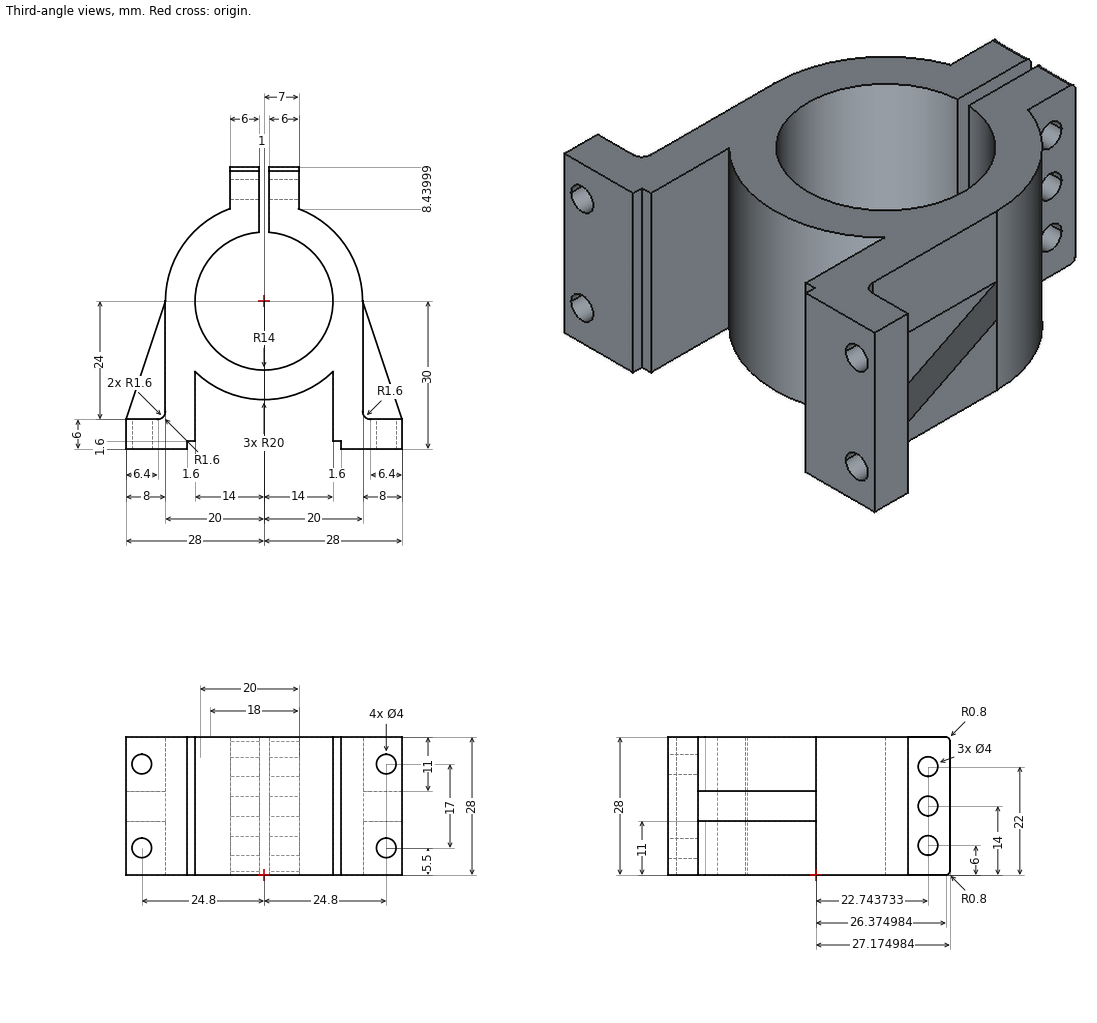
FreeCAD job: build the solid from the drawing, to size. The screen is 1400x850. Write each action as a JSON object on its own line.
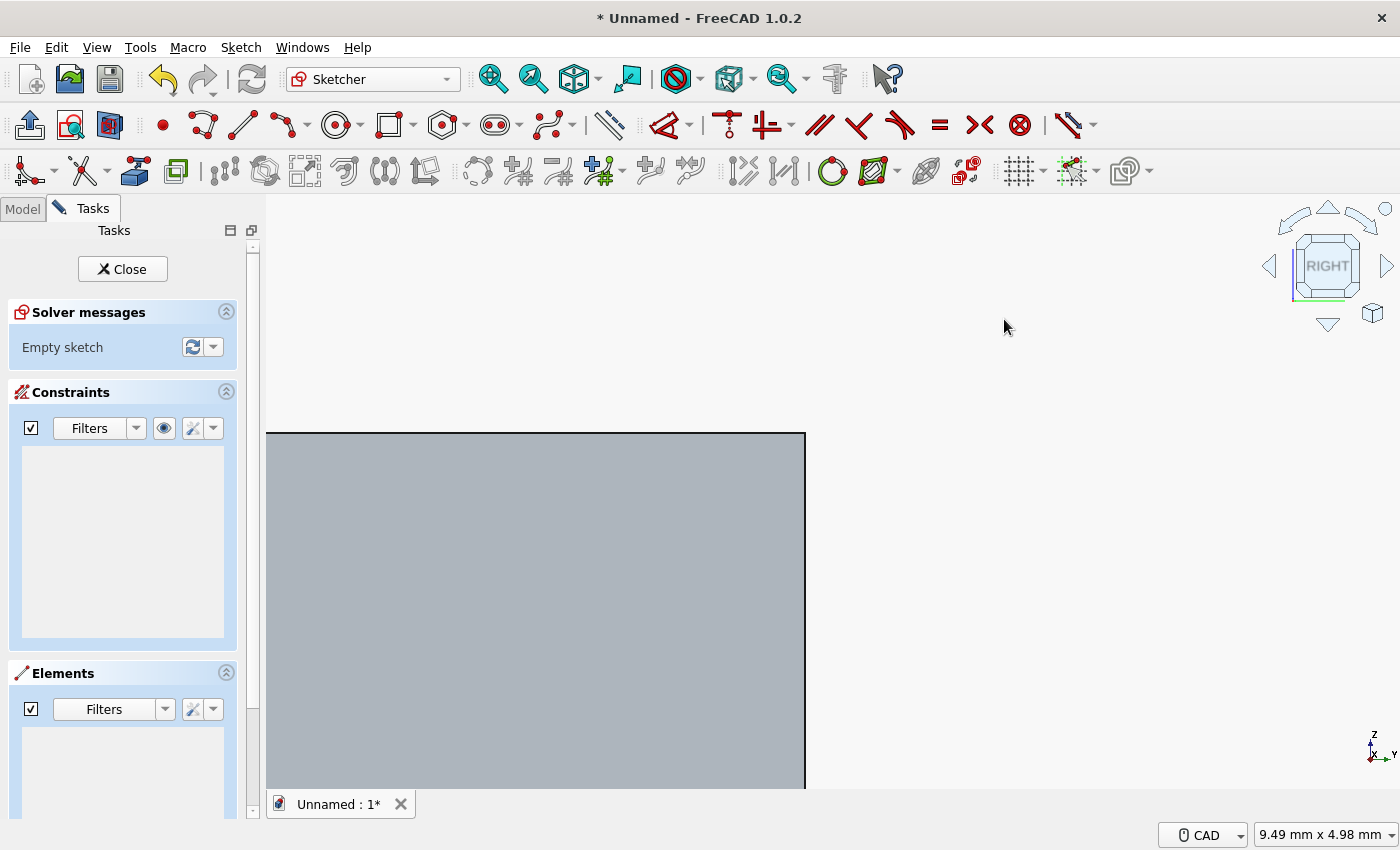
{"action": "scroll", "coordinate": [754, 478], "scroll_direction": "up", "scroll_amount": 7}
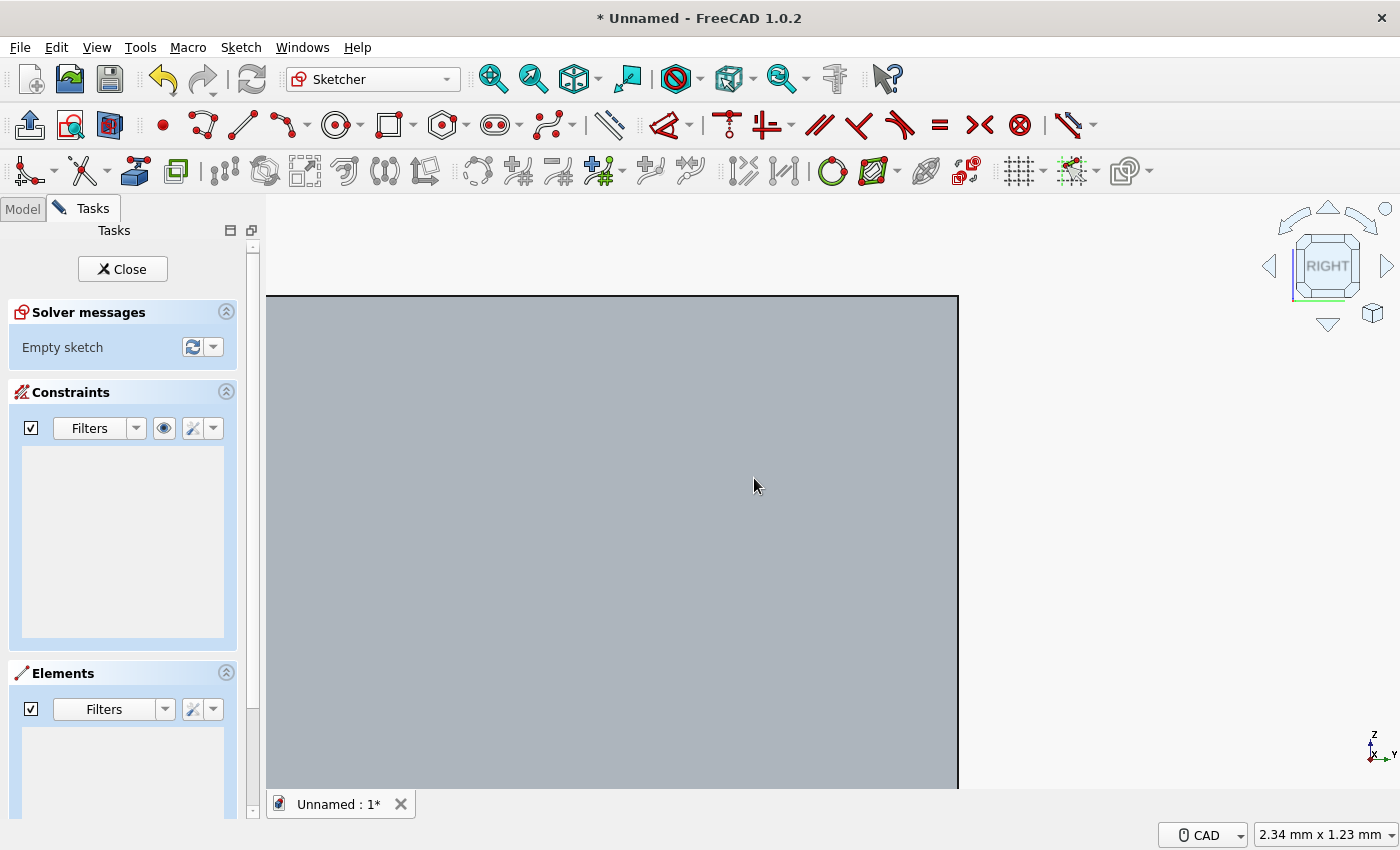
{"action": "left_click", "coordinate": [204, 126]}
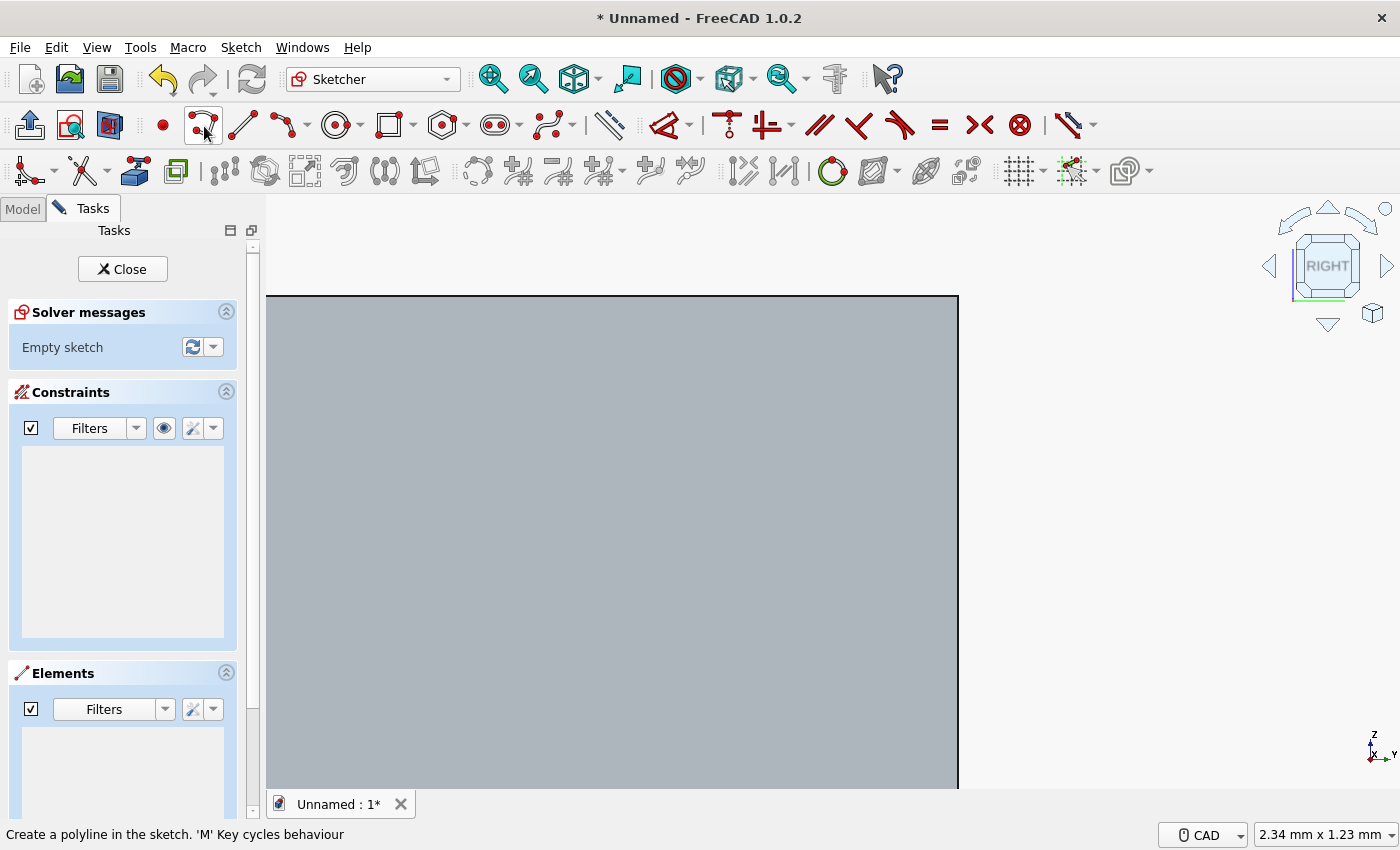
{"action": "left_click", "coordinate": [958, 684]}
{"action": "left_click", "coordinate": [958, 296]}
{"action": "left_click", "coordinate": [570, 296]}
{"action": "right_click", "coordinate": [570, 296]}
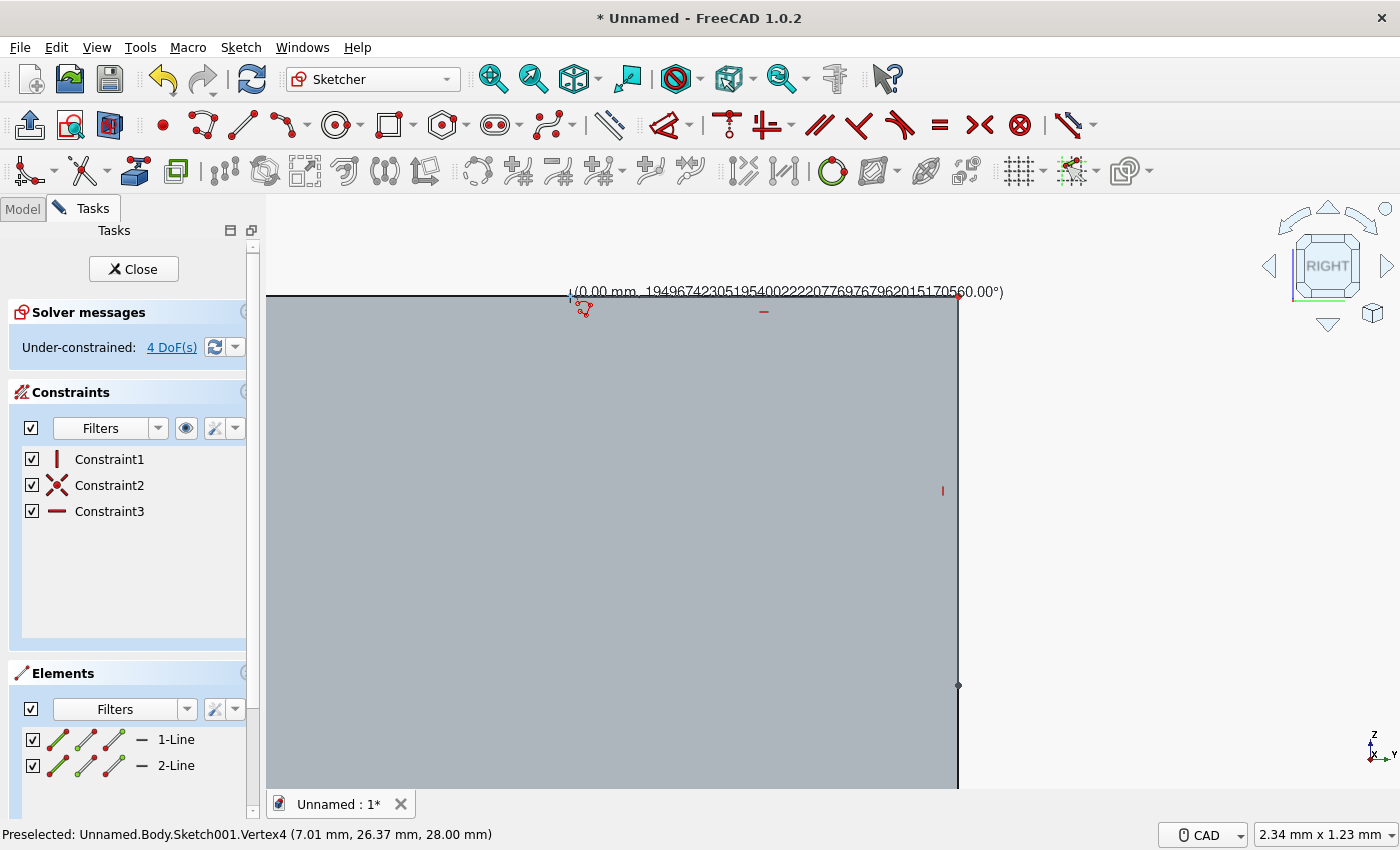
{"action": "left_click", "coordinate": [284, 126]}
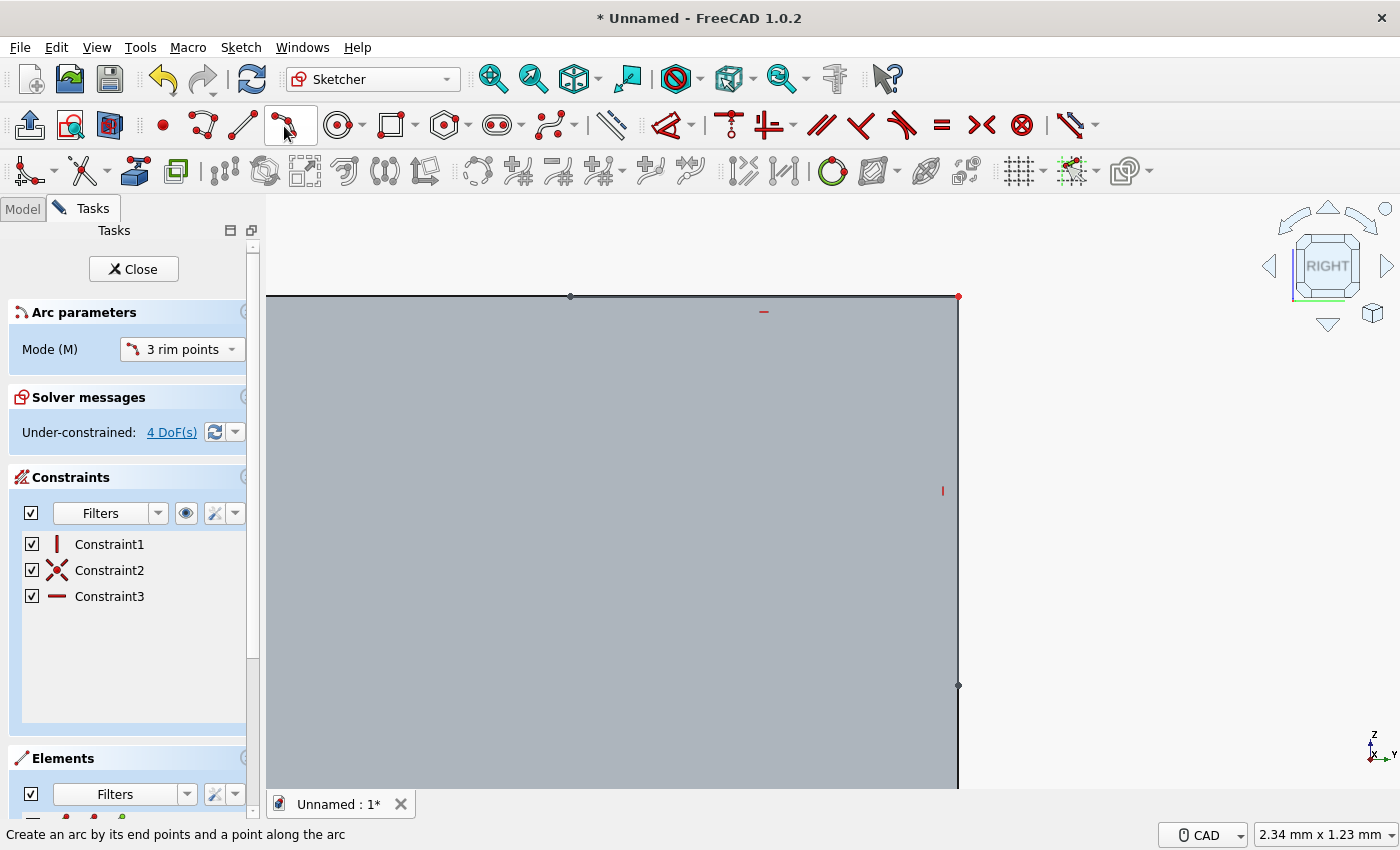
{"action": "left_click", "coordinate": [570, 297]}
{"action": "left_click", "coordinate": [958, 685]}
{"action": "left_click", "coordinate": [844, 410]}
{"action": "key", "text": "Escape"}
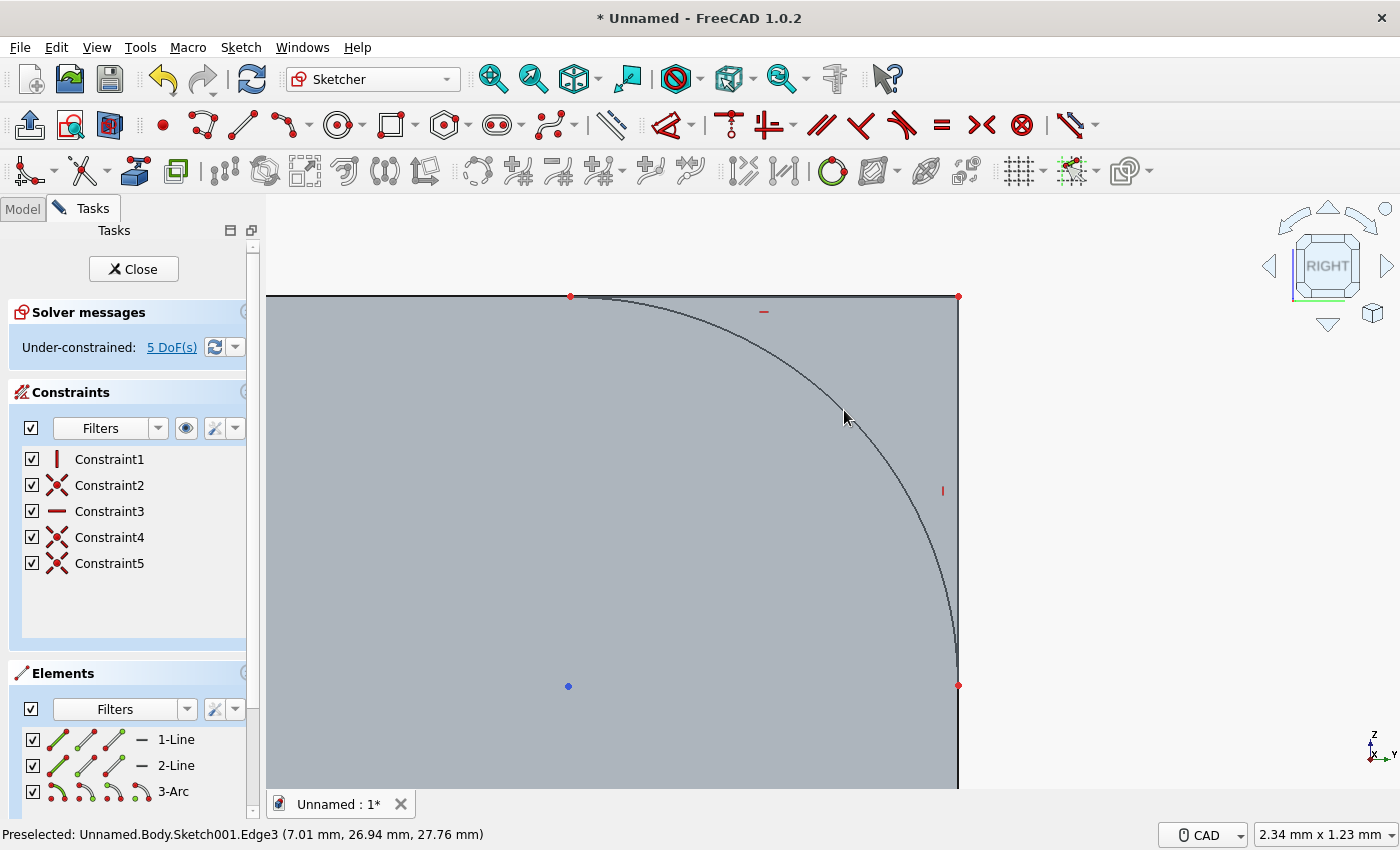
{"action": "left_click", "coordinate": [958, 569]}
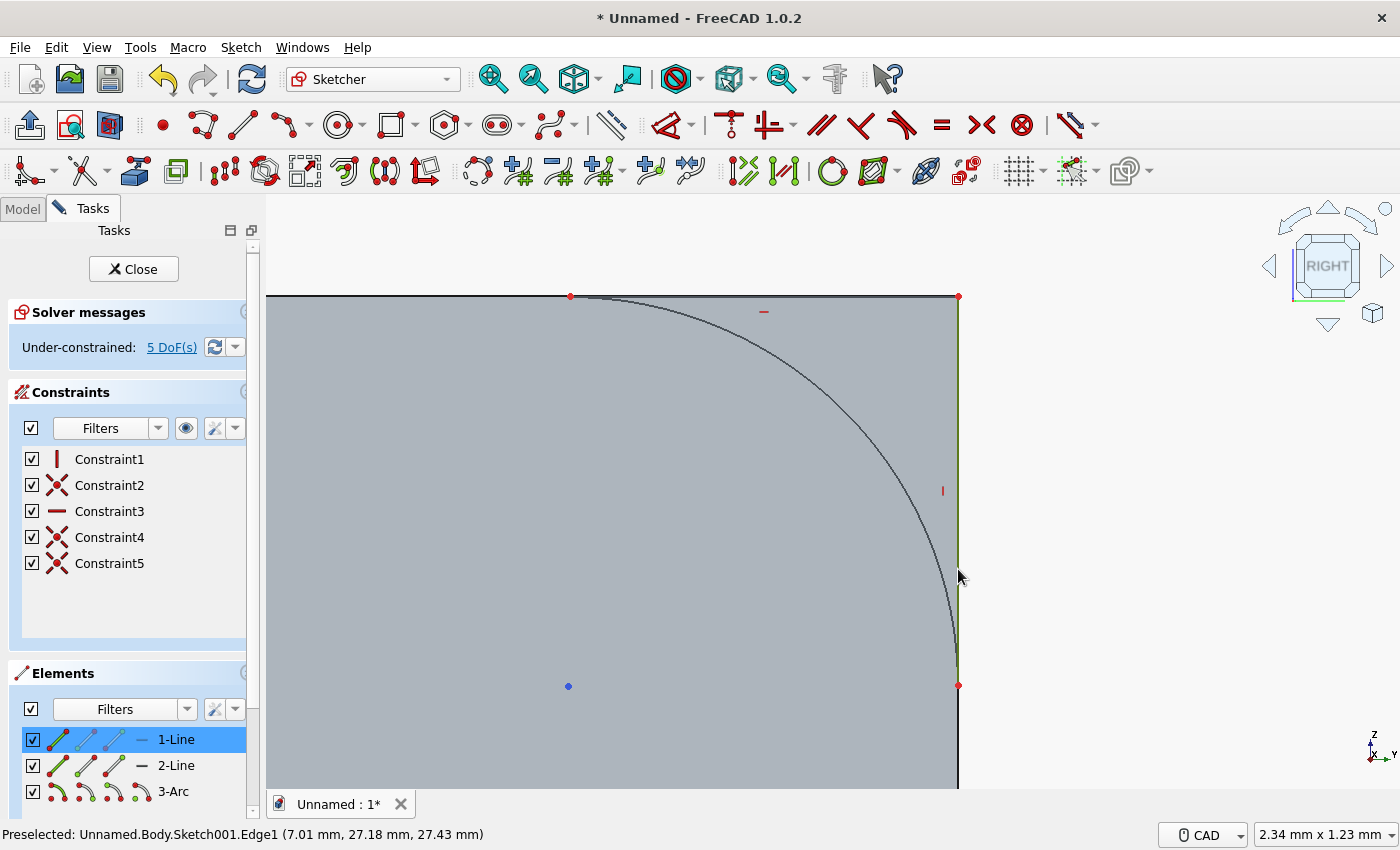
{"action": "left_click", "coordinate": [915, 509]}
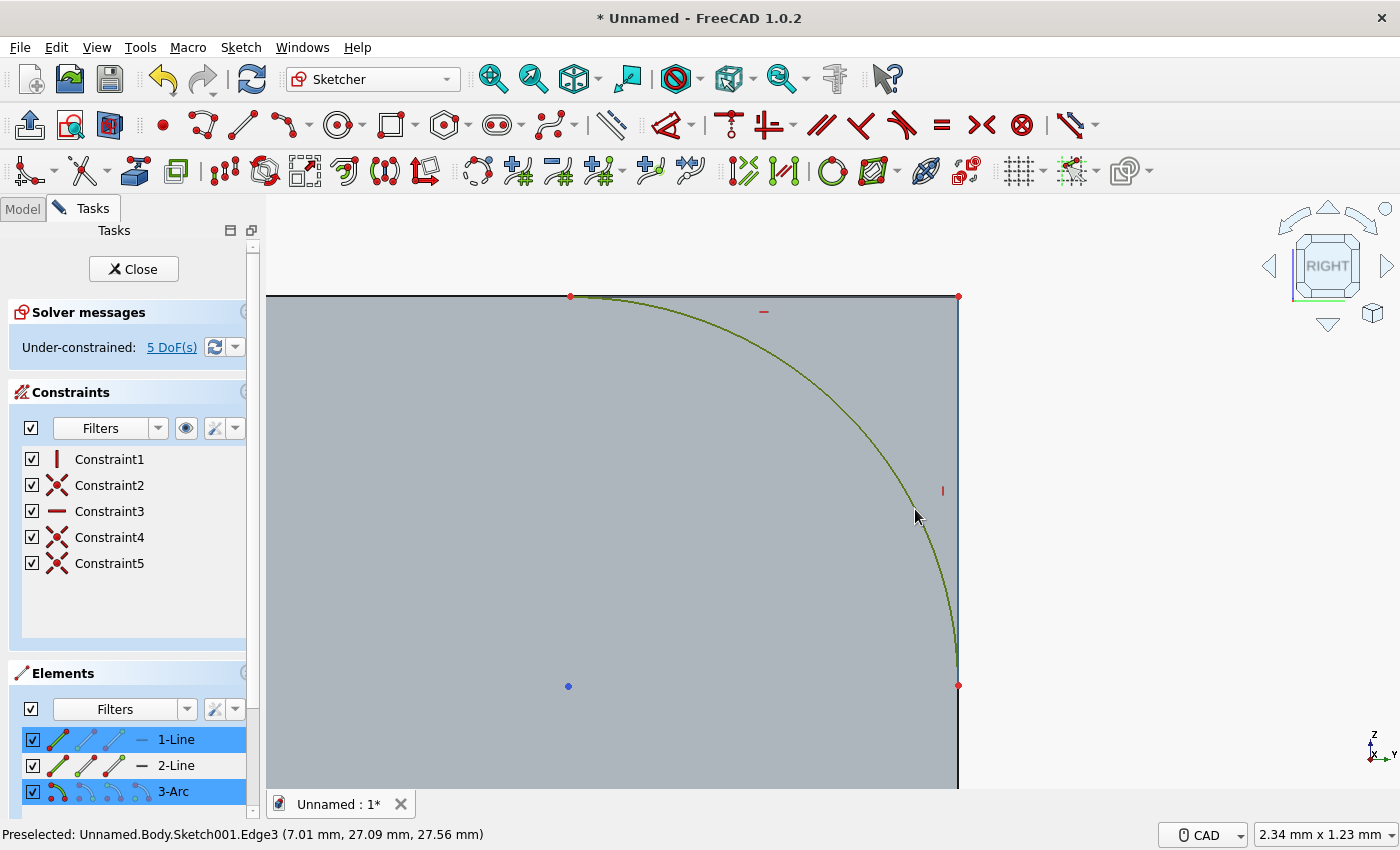
{"action": "left_click", "coordinate": [902, 126]}